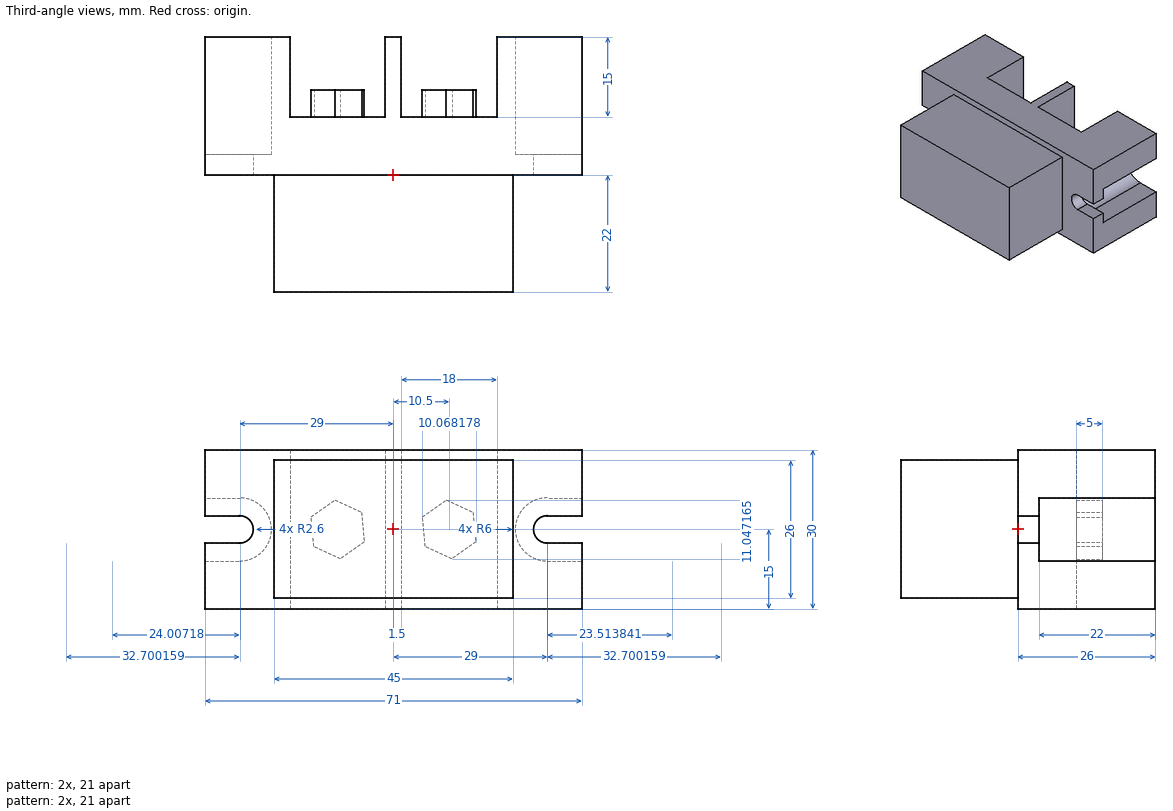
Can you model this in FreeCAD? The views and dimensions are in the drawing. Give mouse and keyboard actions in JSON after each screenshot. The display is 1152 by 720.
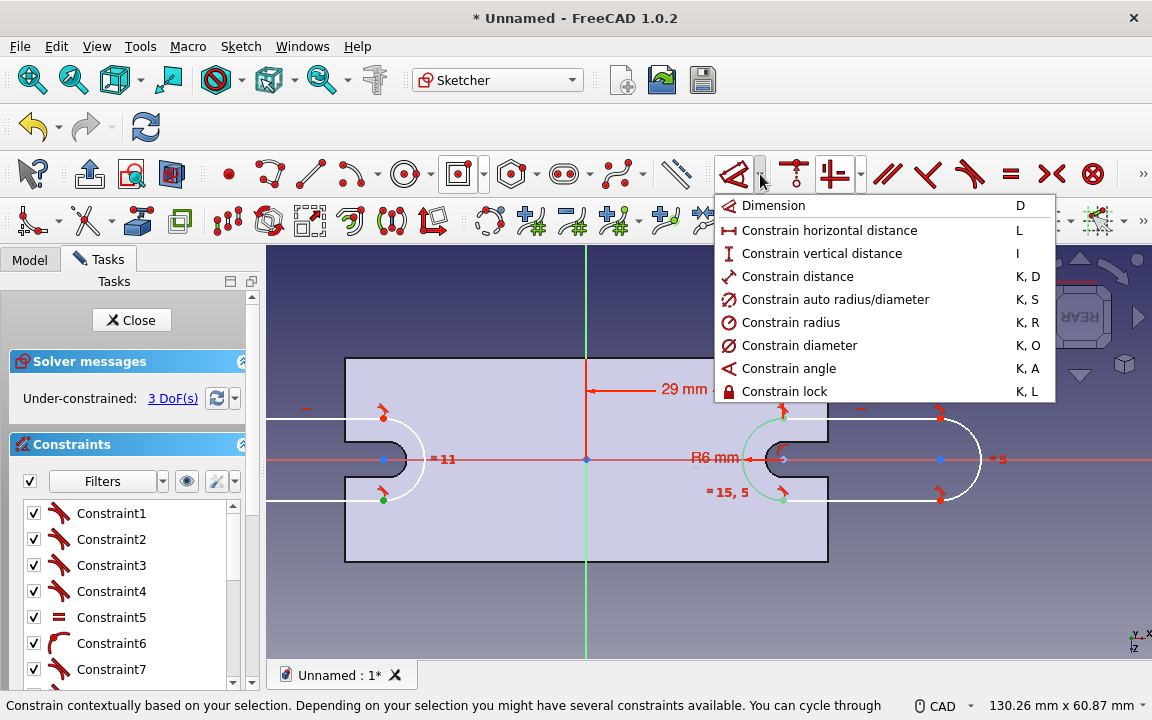
{"action": "left_click", "coordinate": [885, 230]}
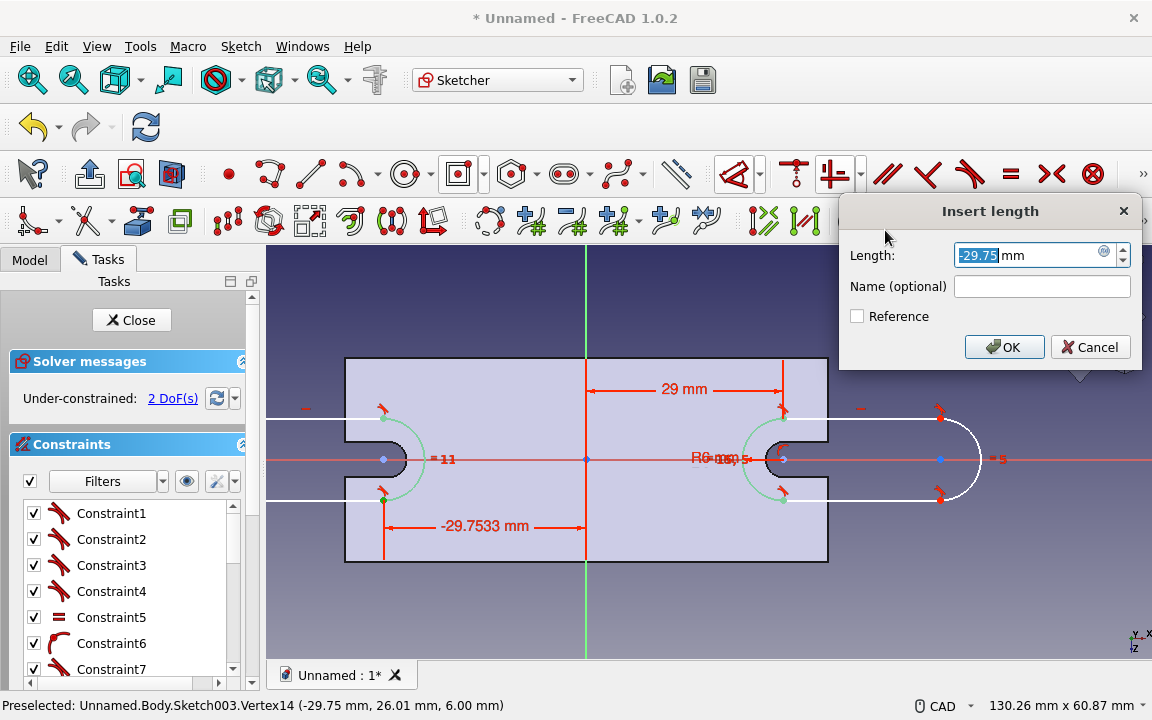
{"action": "type", "text": "-29"}
{"action": "key", "text": "Return"}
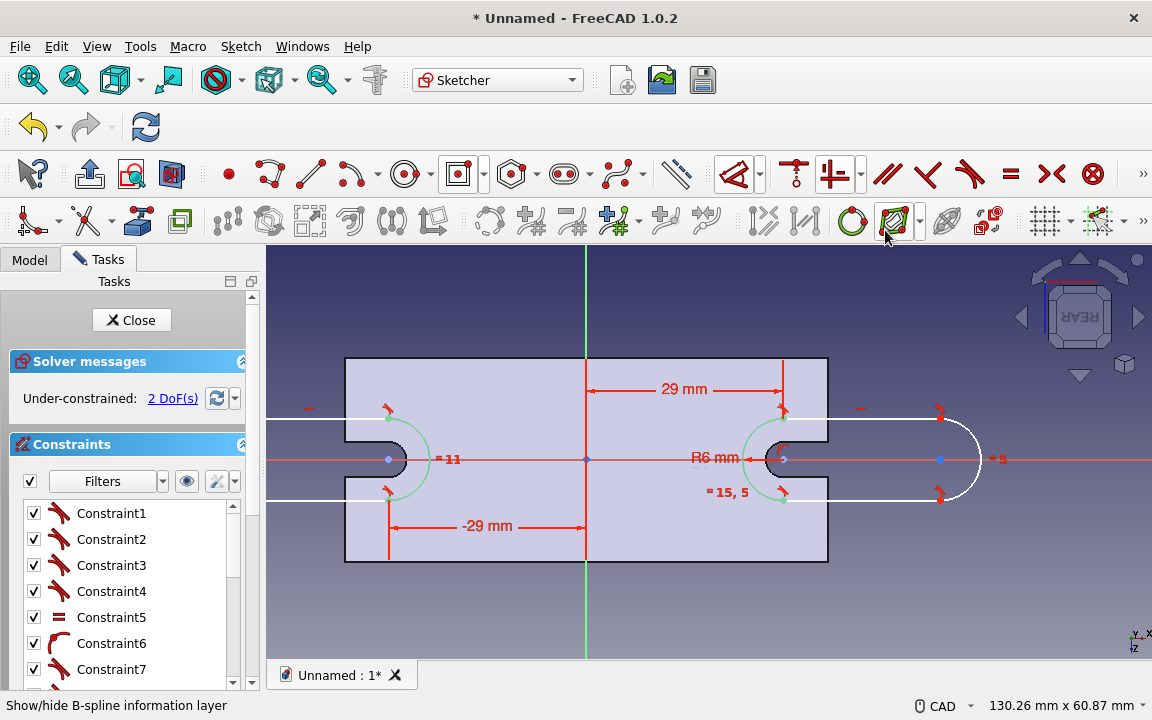
{"action": "left_click", "coordinate": [341, 419]}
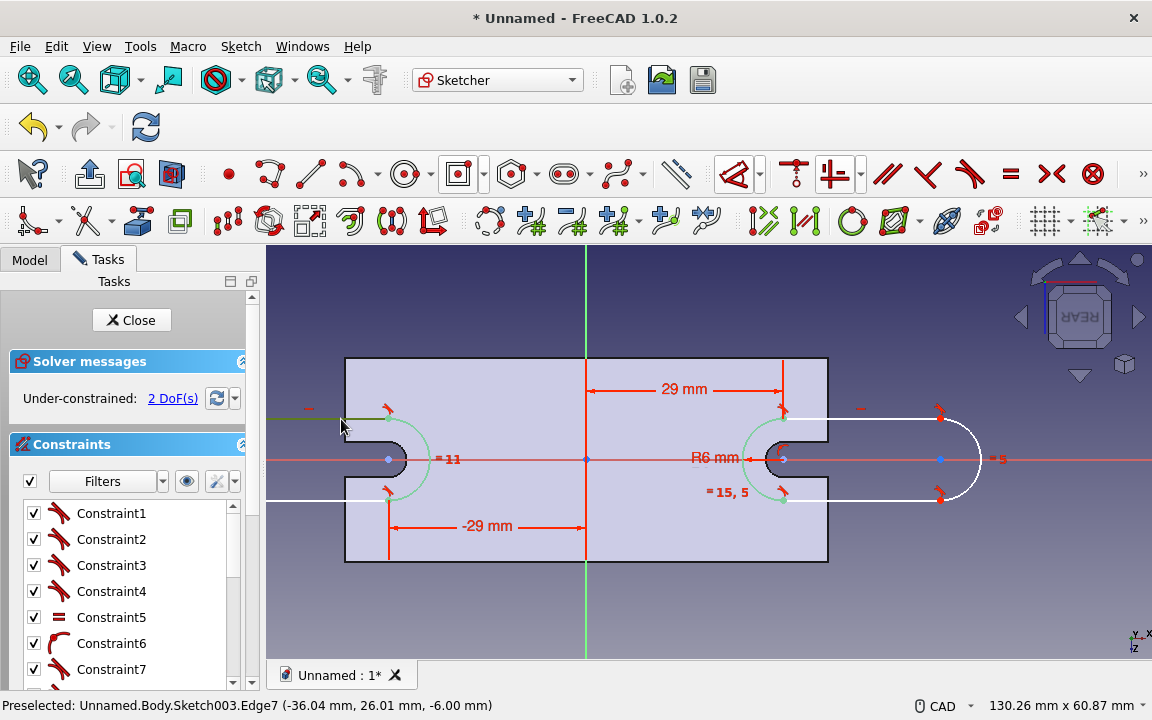
{"action": "key", "text": "l"}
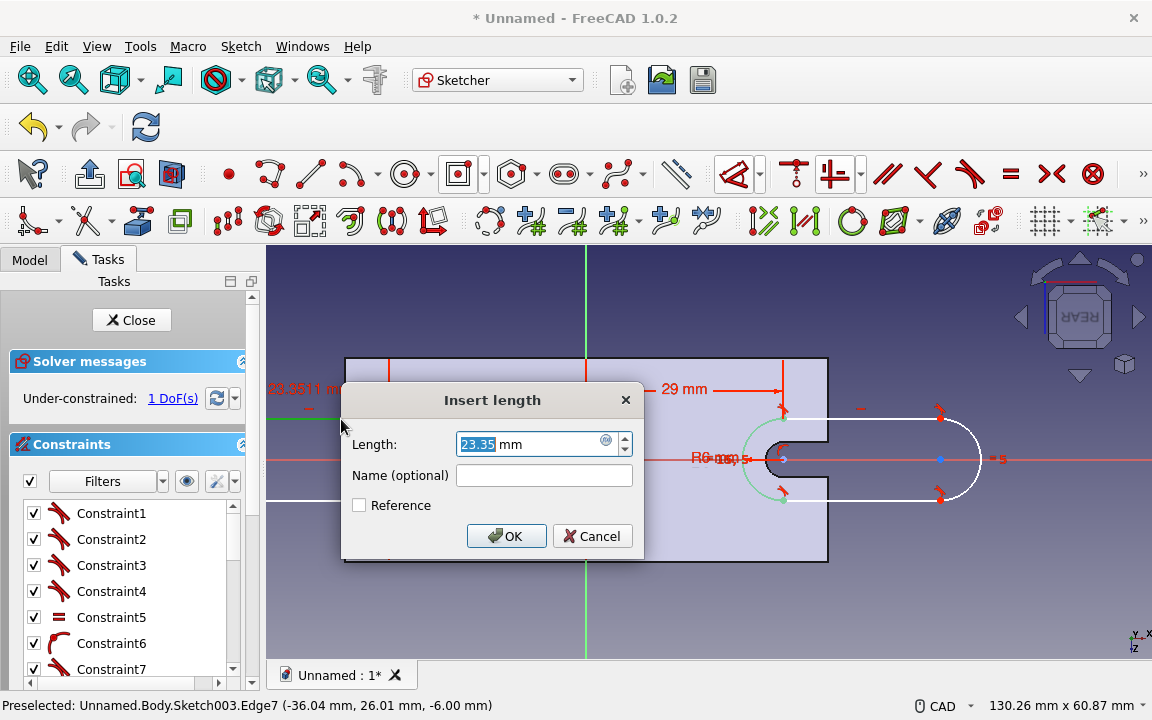
{"action": "type", "text": "24.00718"}
{"action": "key", "text": "Return"}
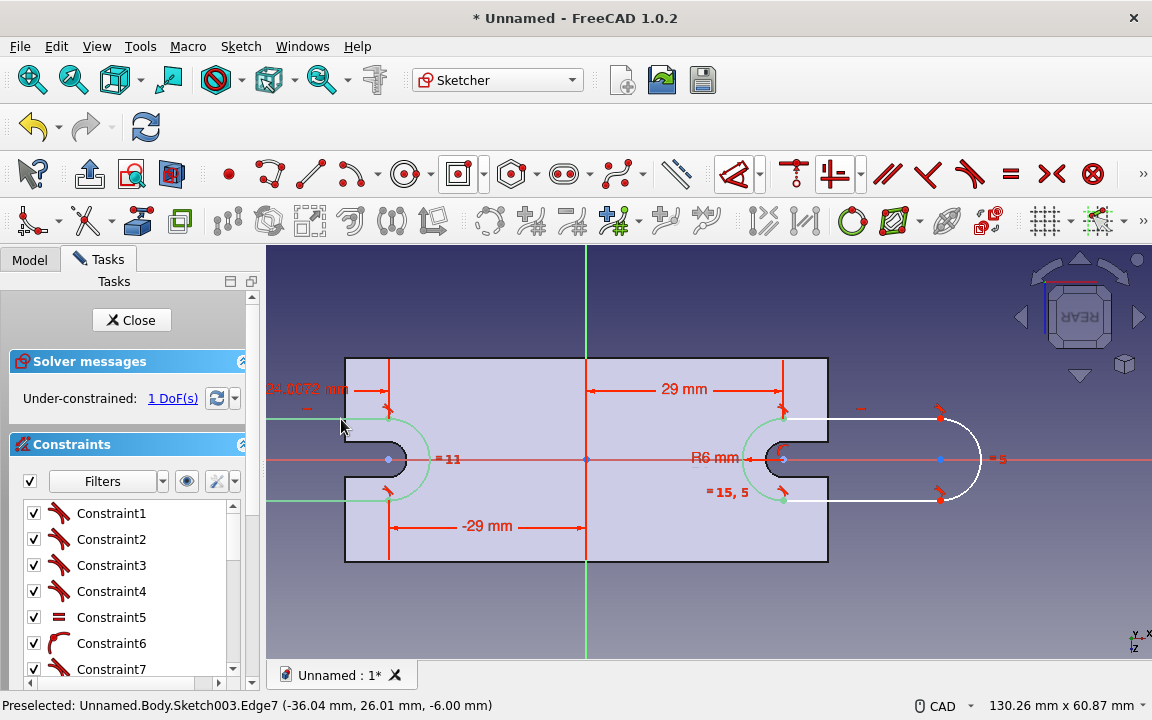
{"action": "left_click", "coordinate": [830, 419]}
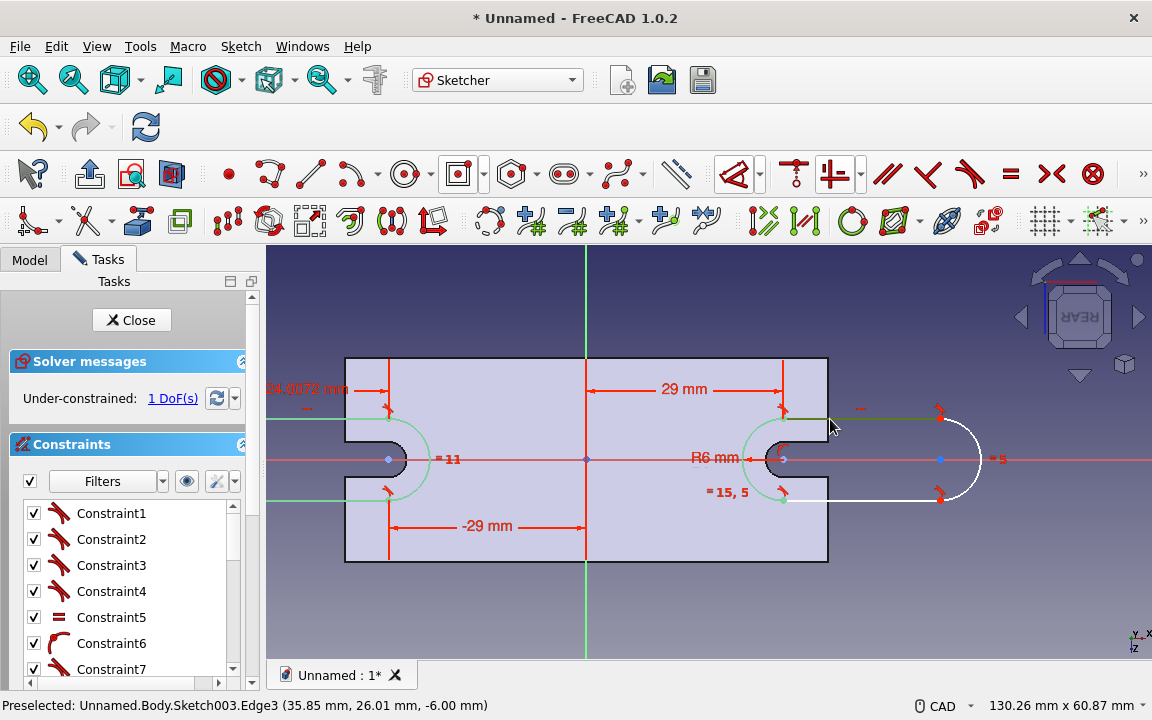
{"action": "key", "text": "l"}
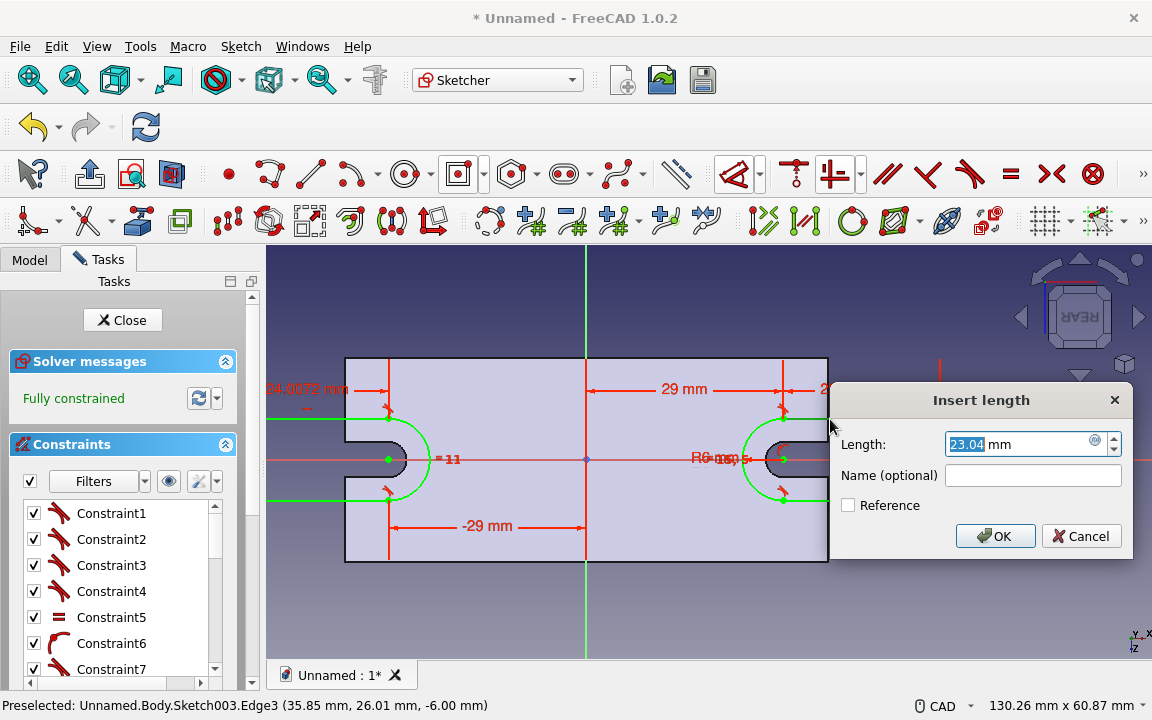
{"action": "type", "text": "23.513841"}
{"action": "key", "text": "Return"}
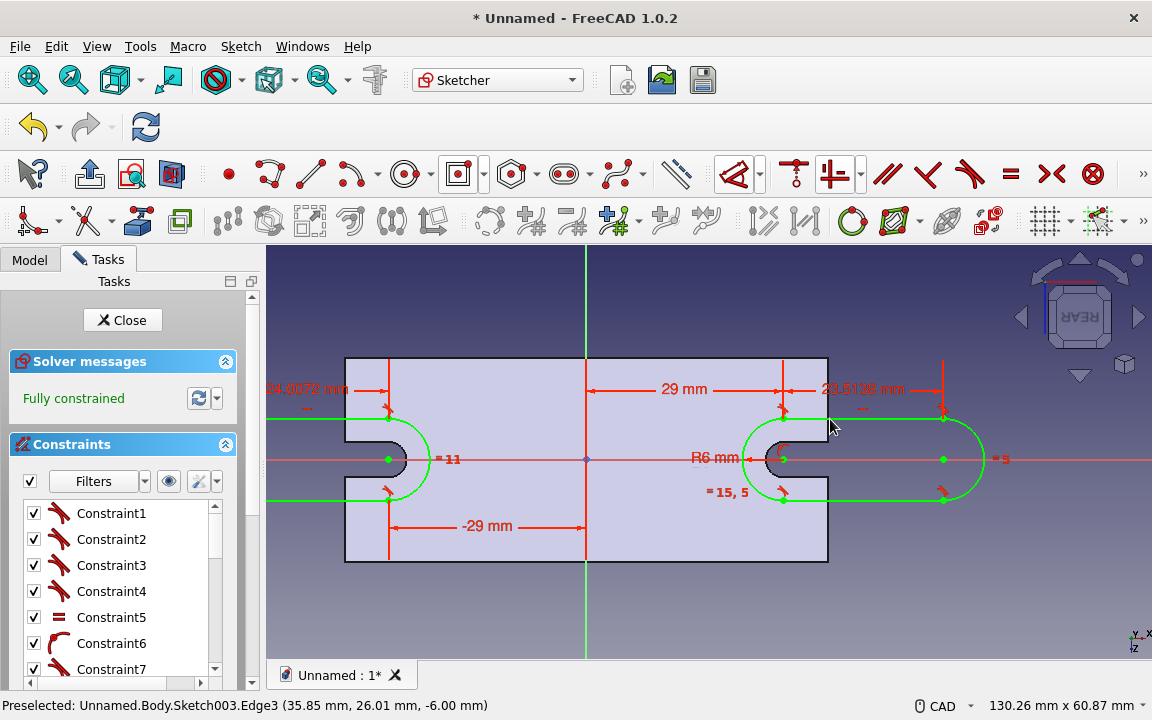
{"action": "left_click", "coordinate": [123, 320]}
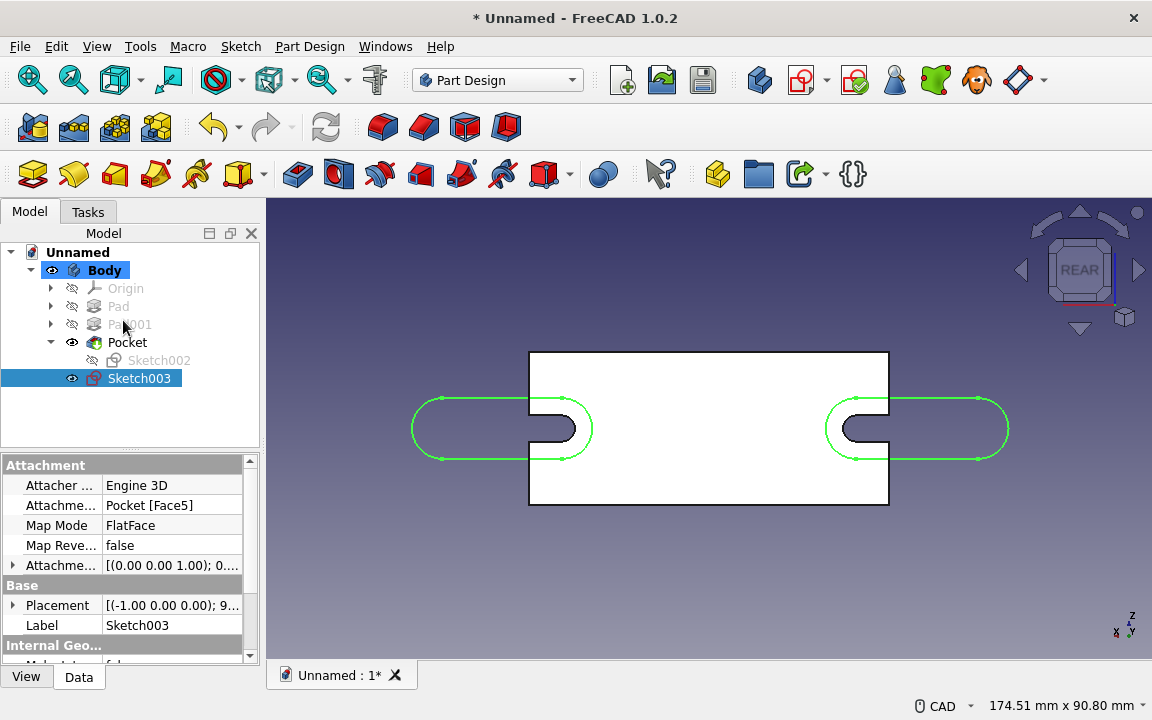
{"action": "left_click", "coordinate": [298, 174]}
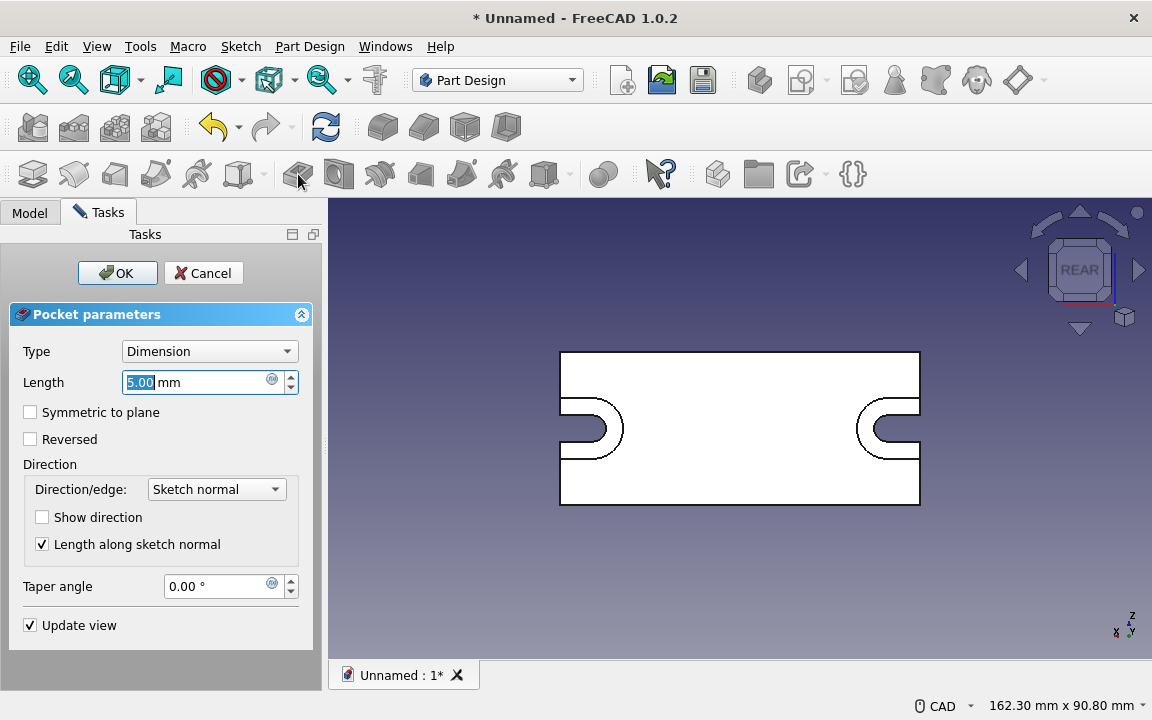
{"action": "type", "text": "22"}
{"action": "key", "text": "Tab"}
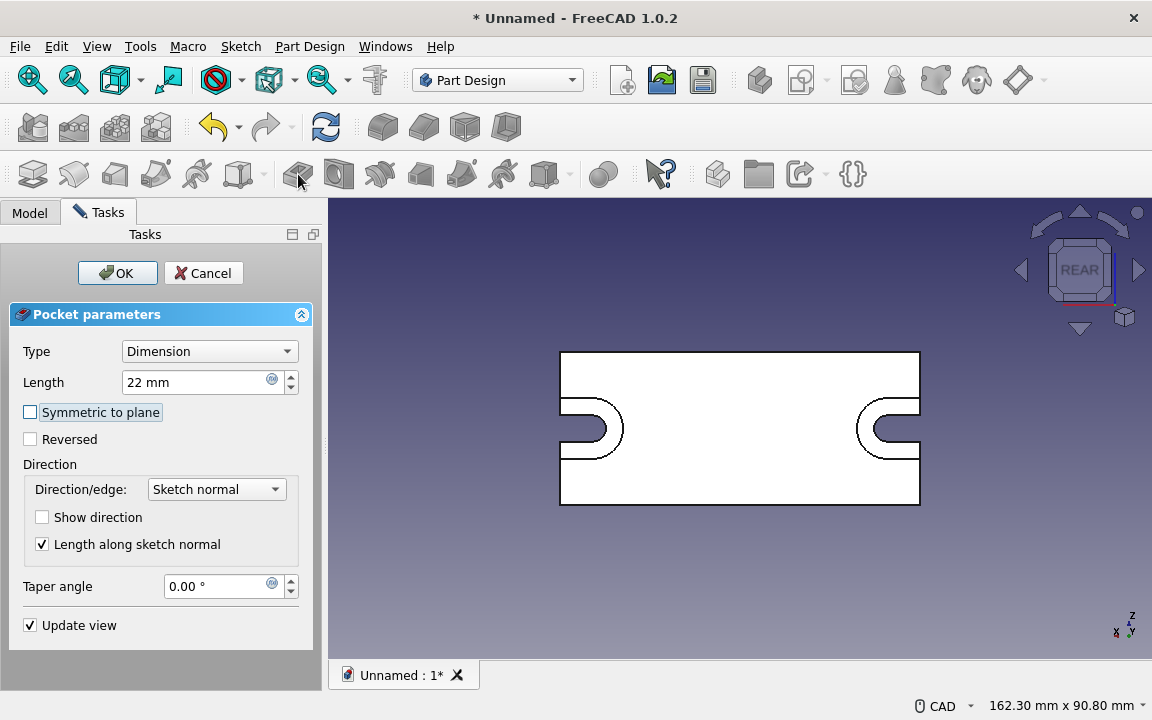
{"action": "left_click", "coordinate": [118, 273]}